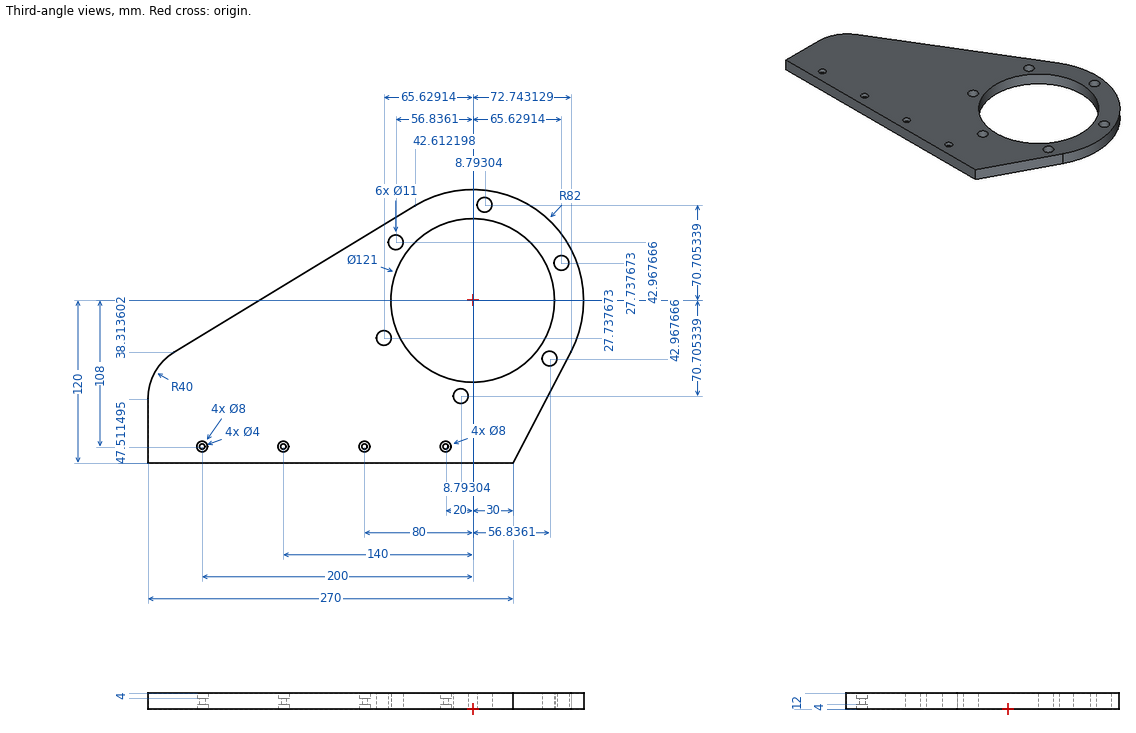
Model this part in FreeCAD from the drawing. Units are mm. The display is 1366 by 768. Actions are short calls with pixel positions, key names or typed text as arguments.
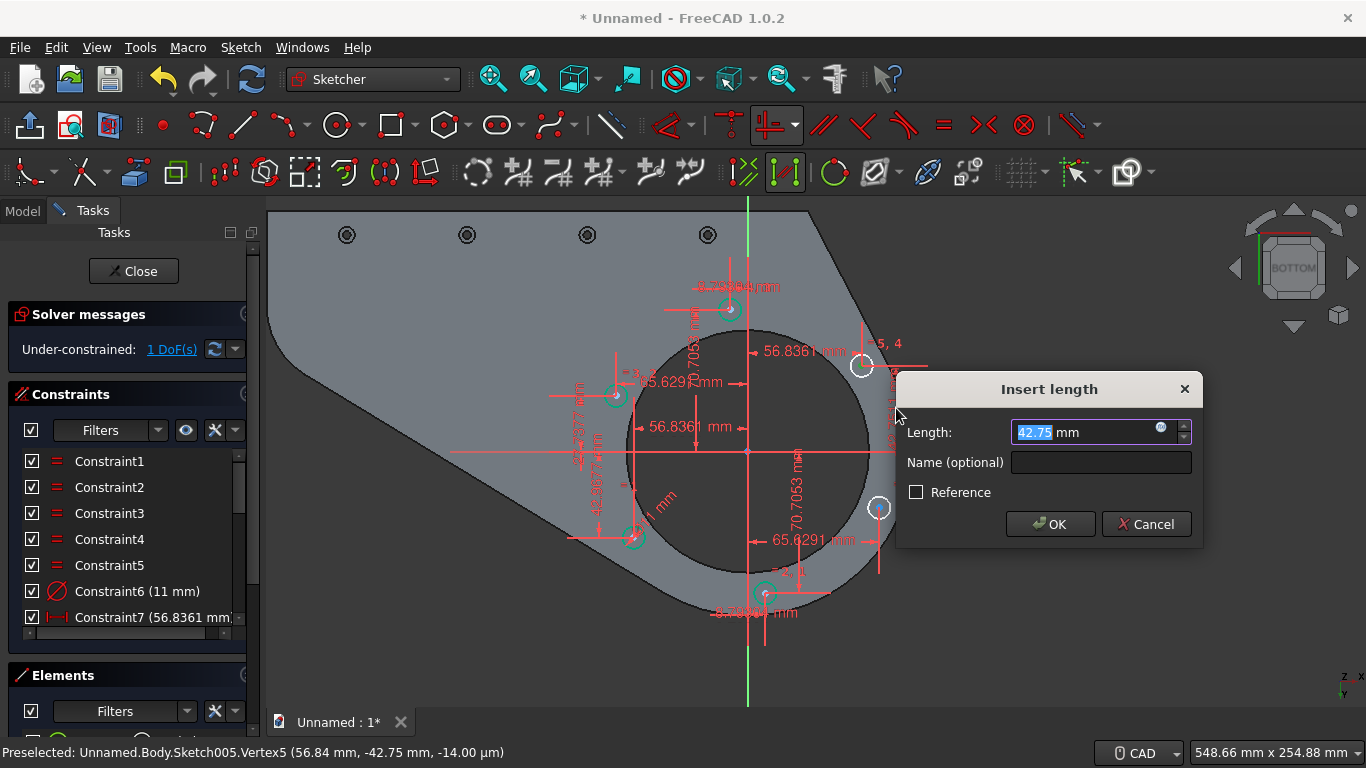
text(42.967666)
key(Return)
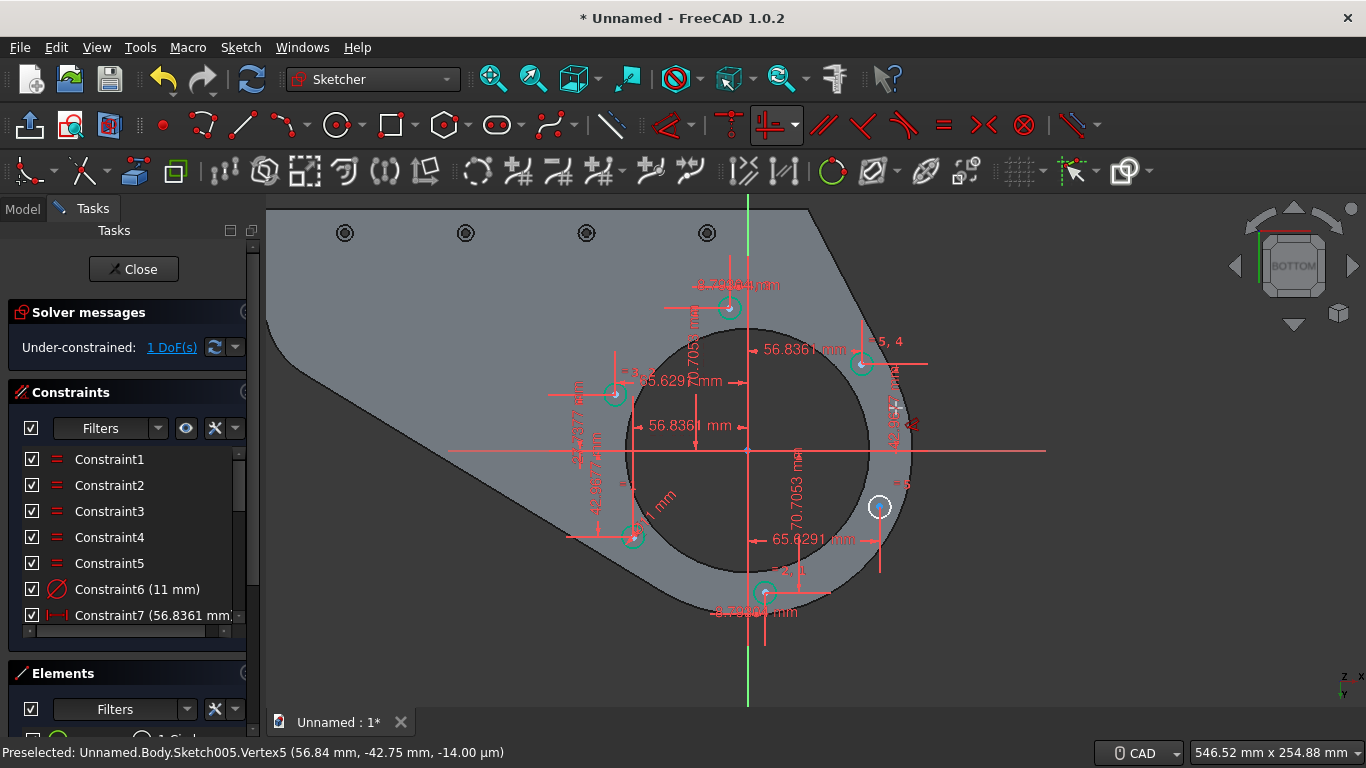
click(880, 507)
click(914, 479)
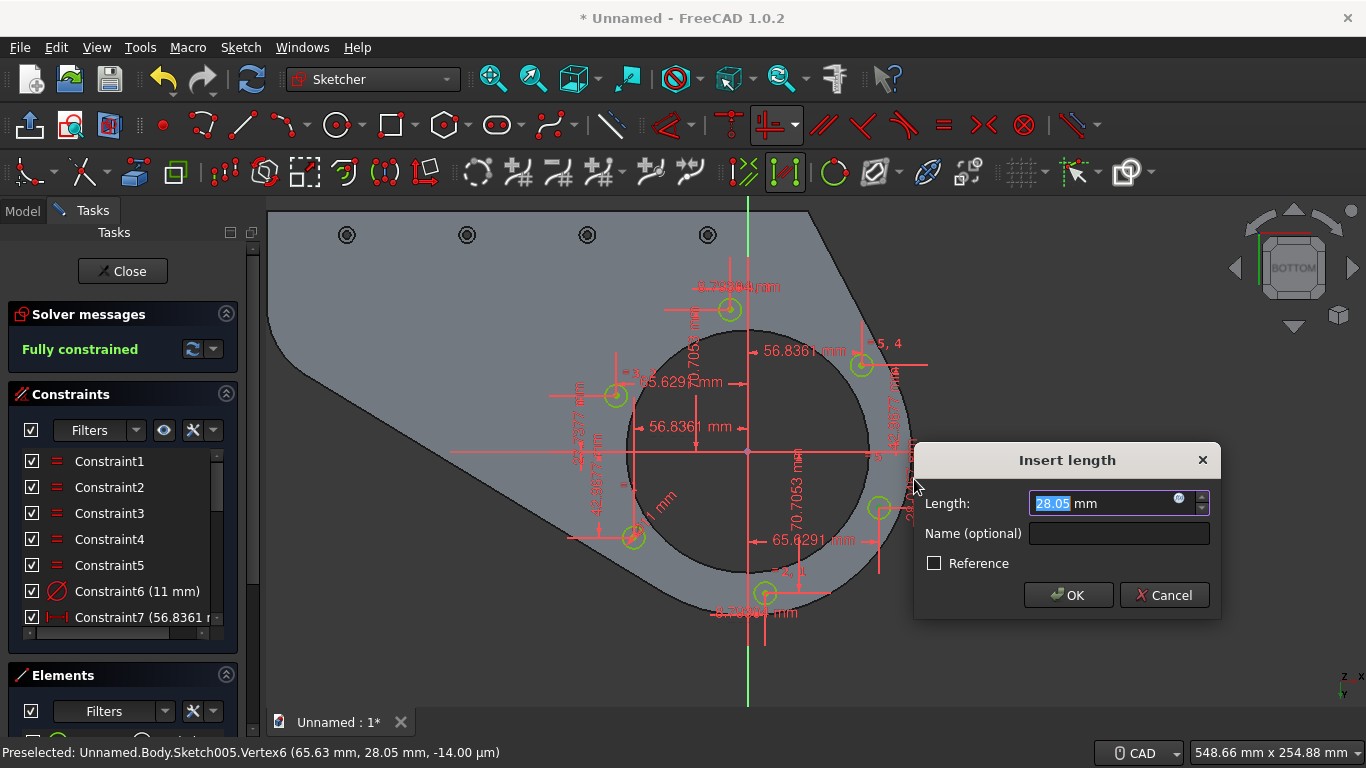
text(27.737673)
key(Return)
key(Escape)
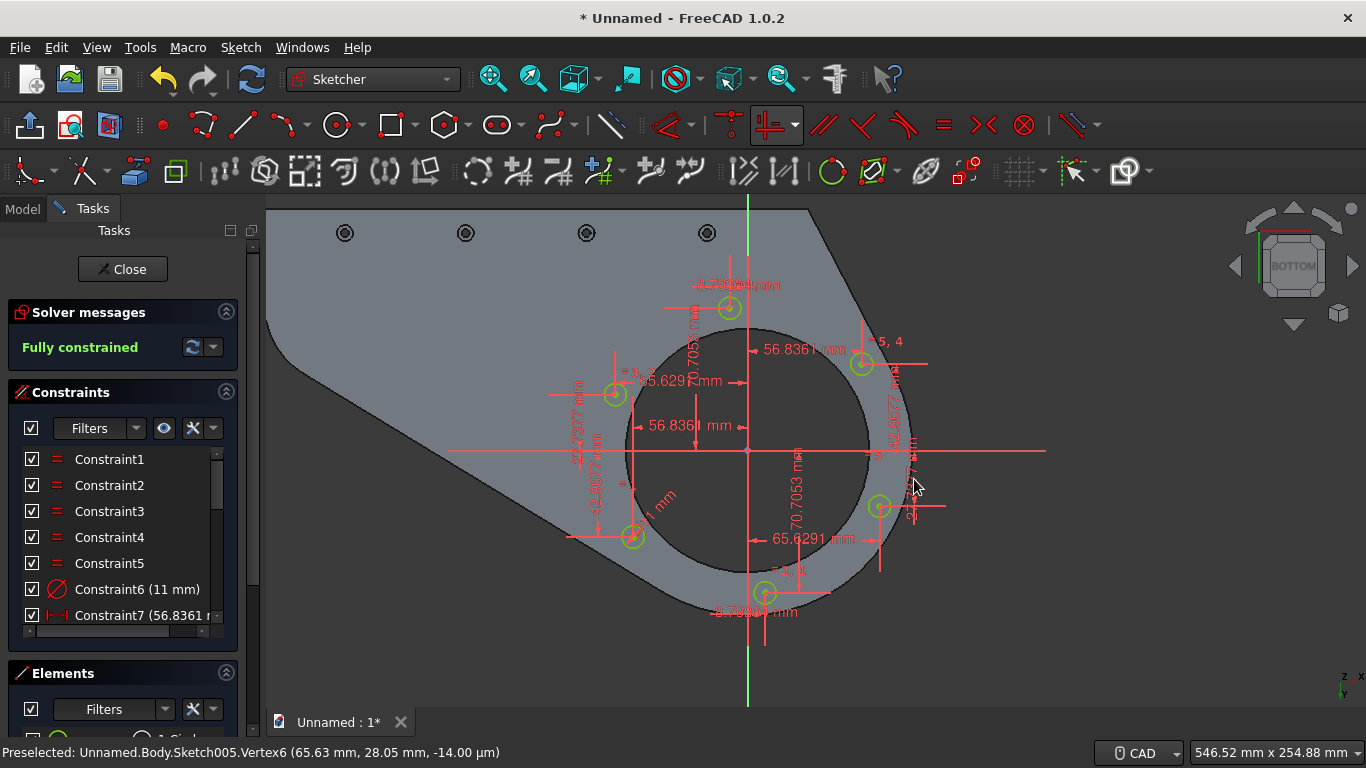
click(123, 269)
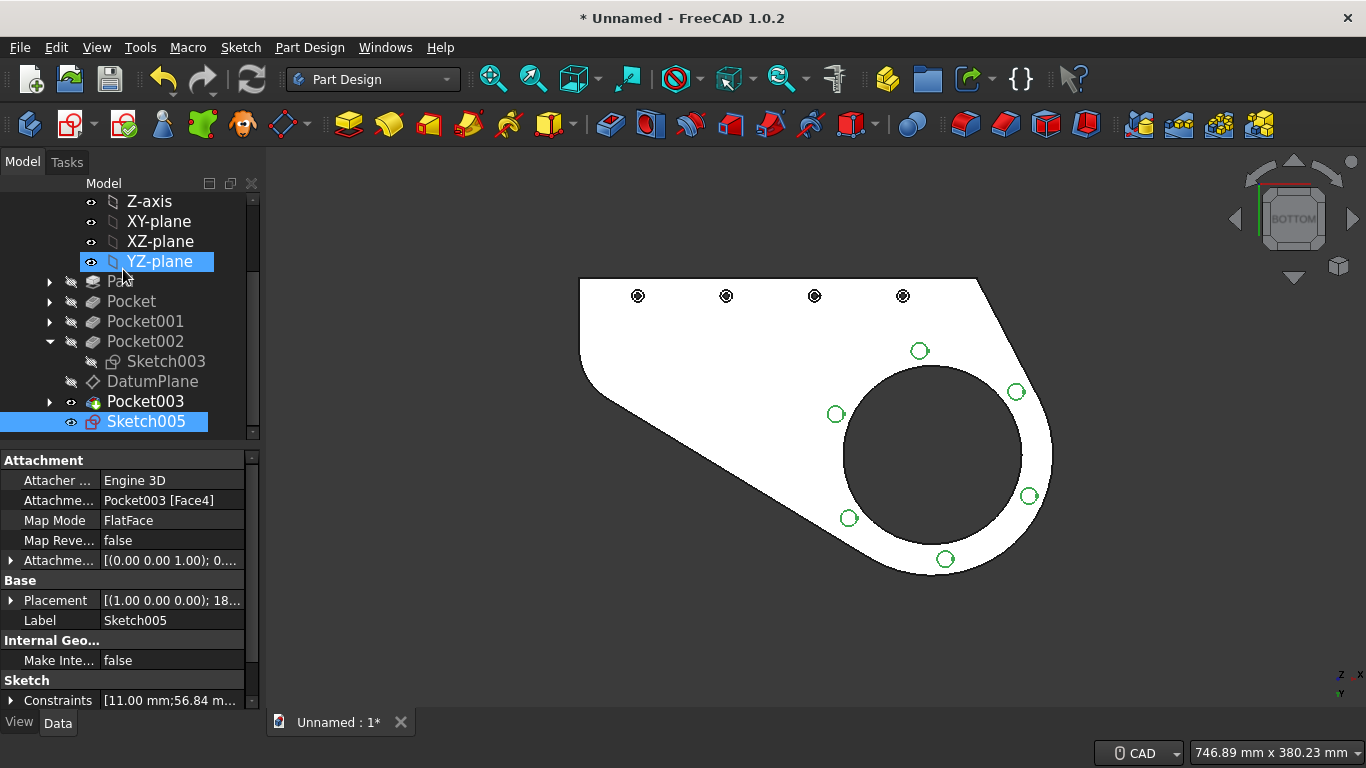
click(612, 124)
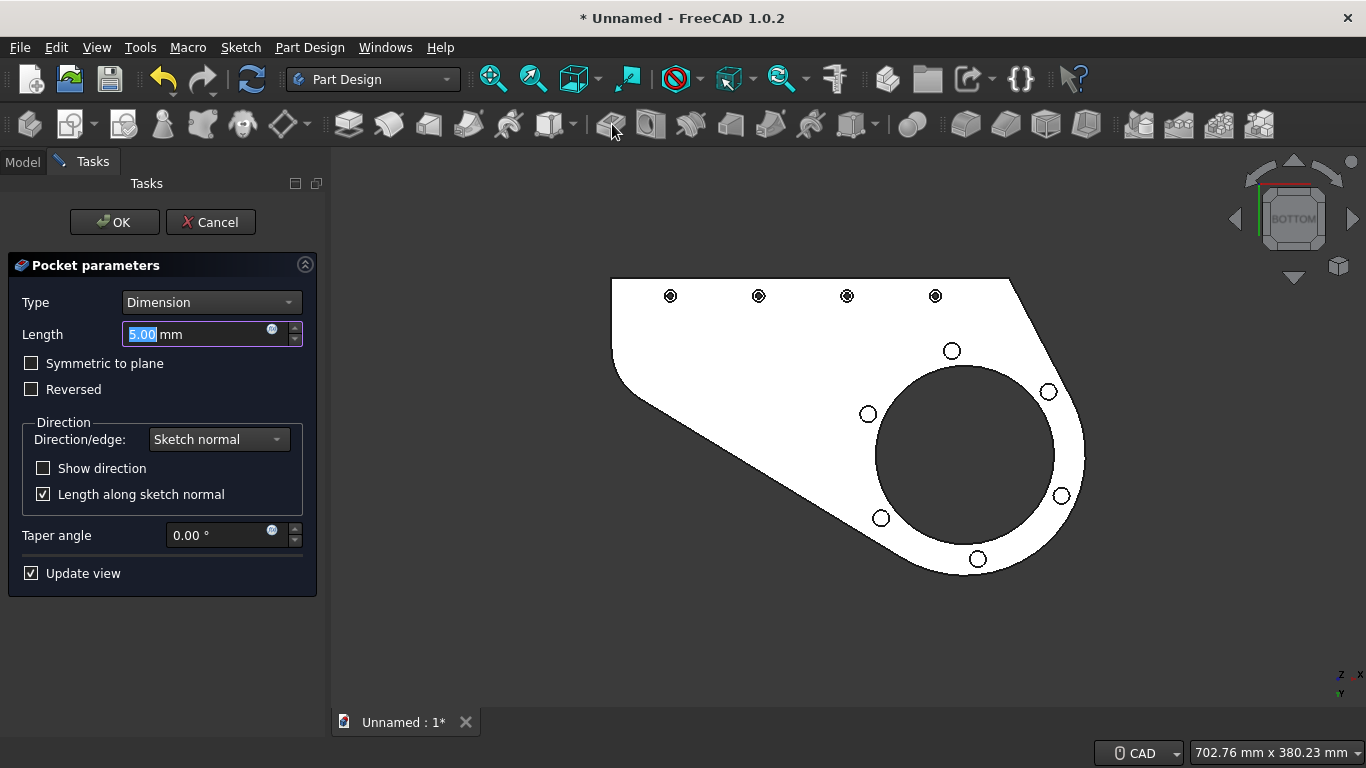
click(212, 302)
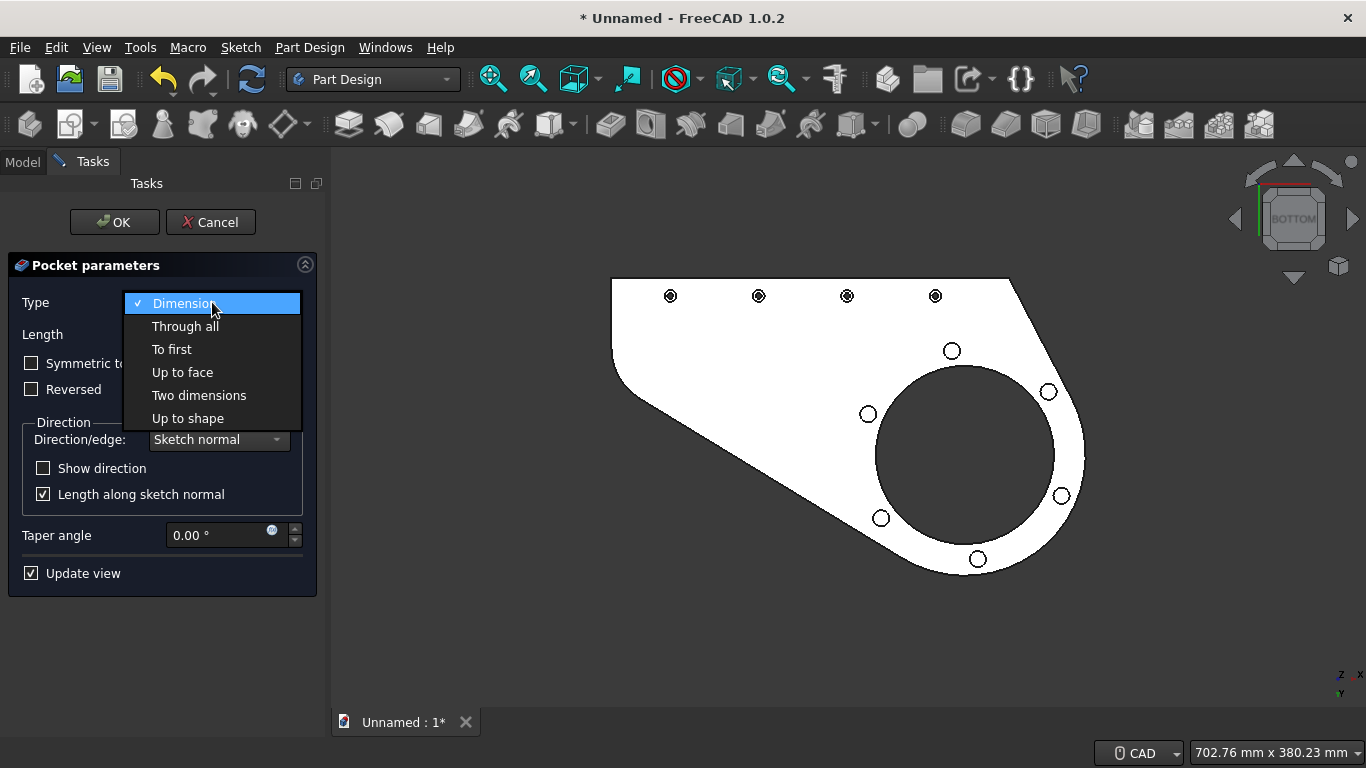
click(212, 326)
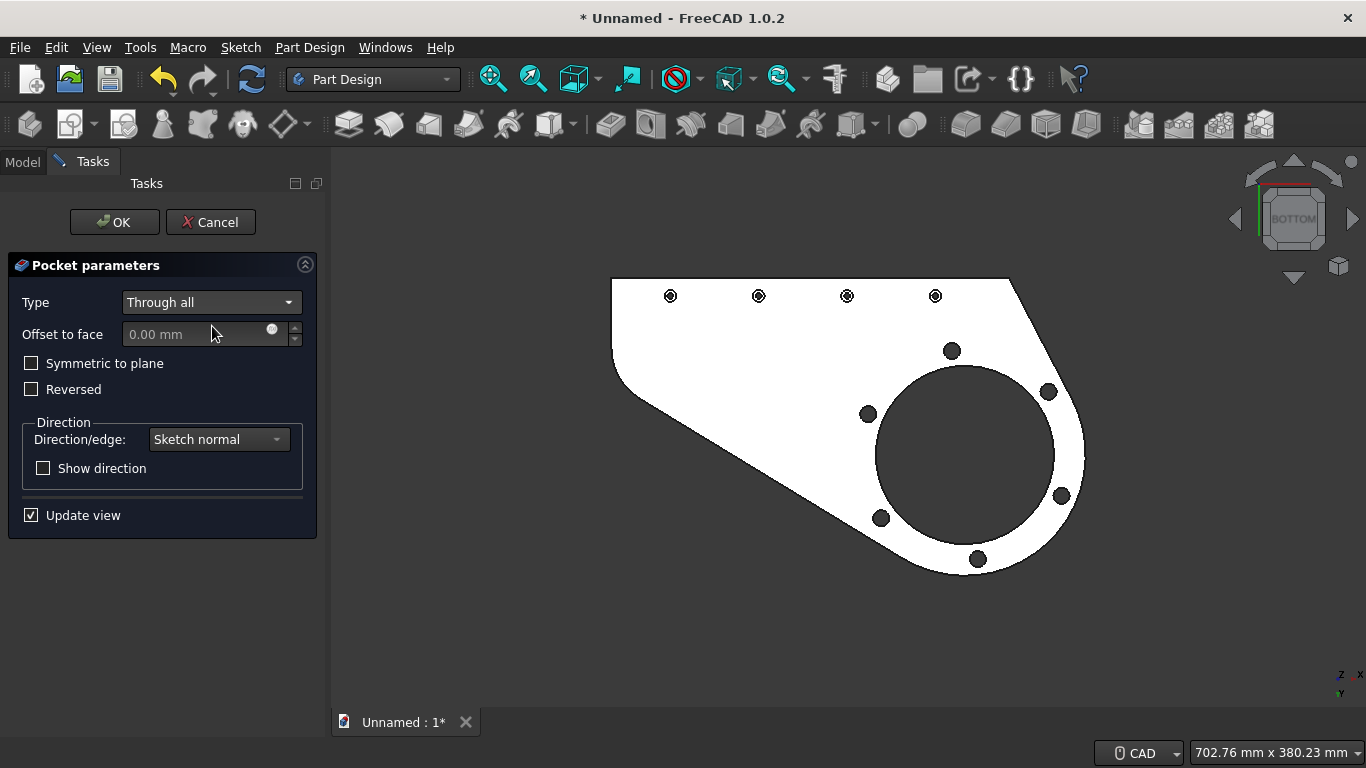
click(115, 222)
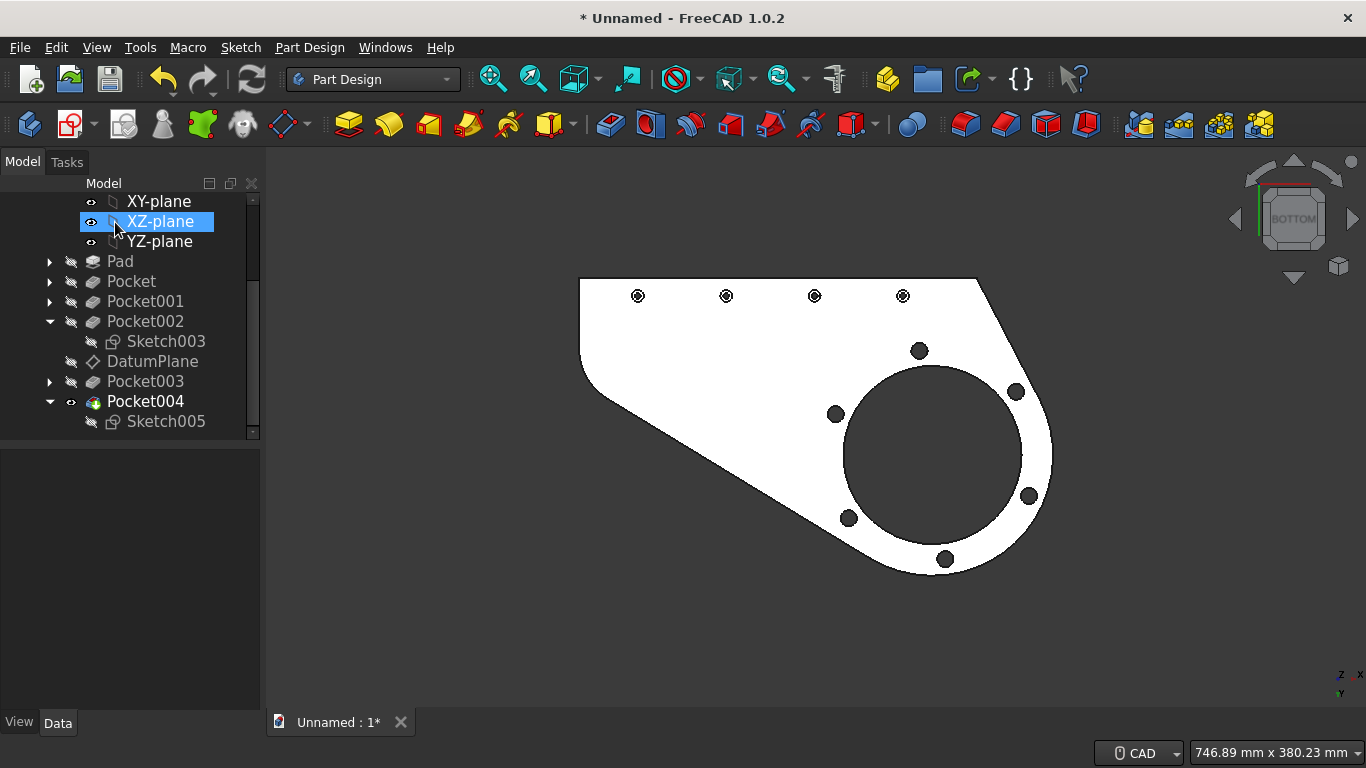
key(0)